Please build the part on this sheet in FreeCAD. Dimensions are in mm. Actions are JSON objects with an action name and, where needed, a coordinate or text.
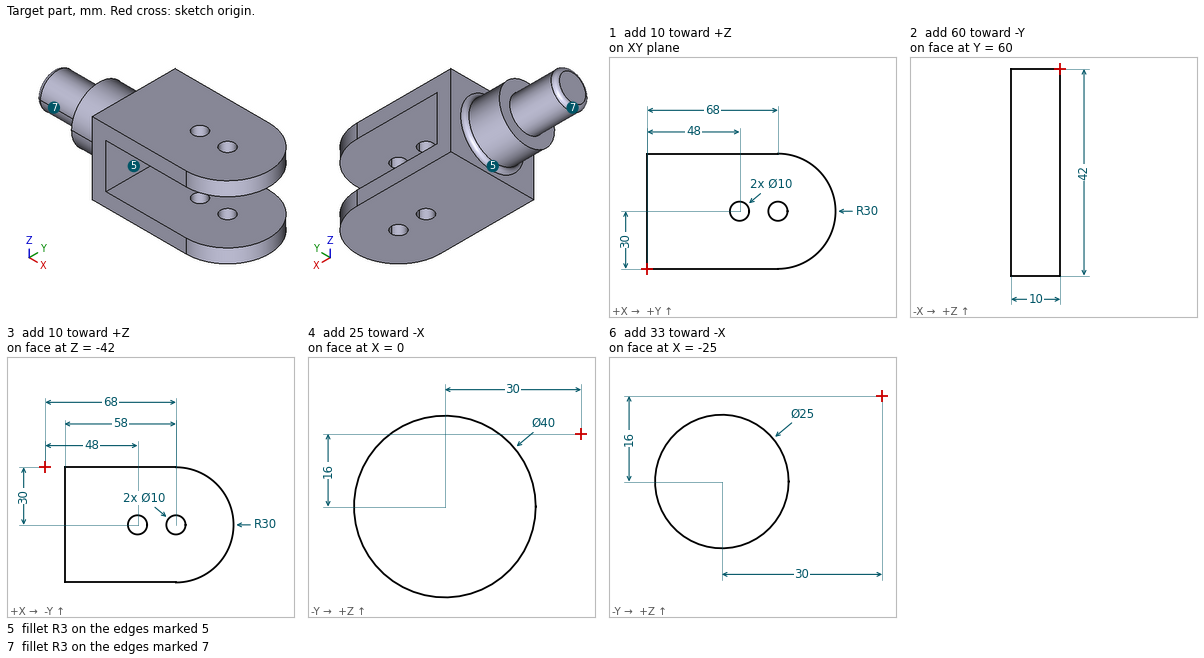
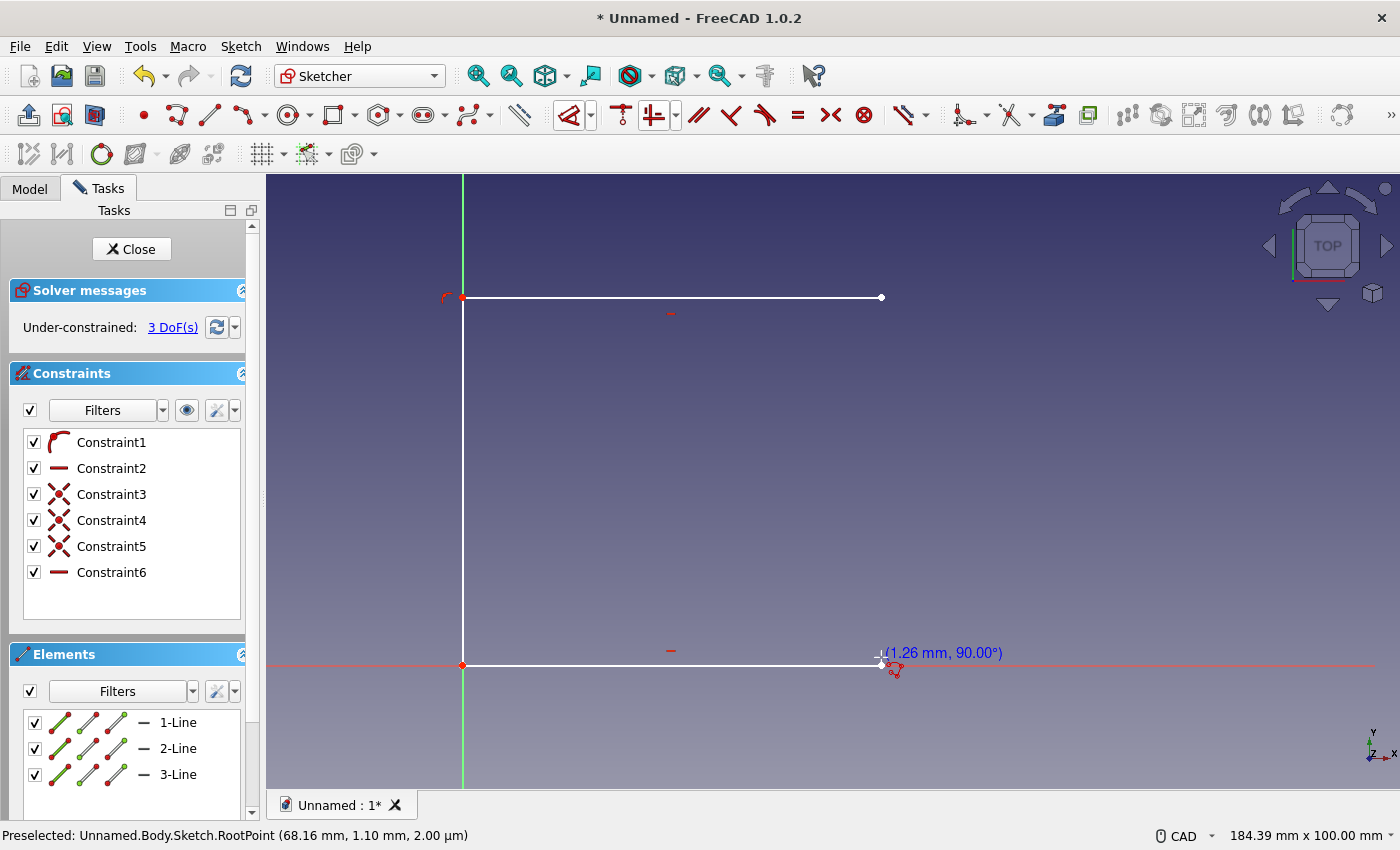
{"action": "key", "text": "g 3 a"}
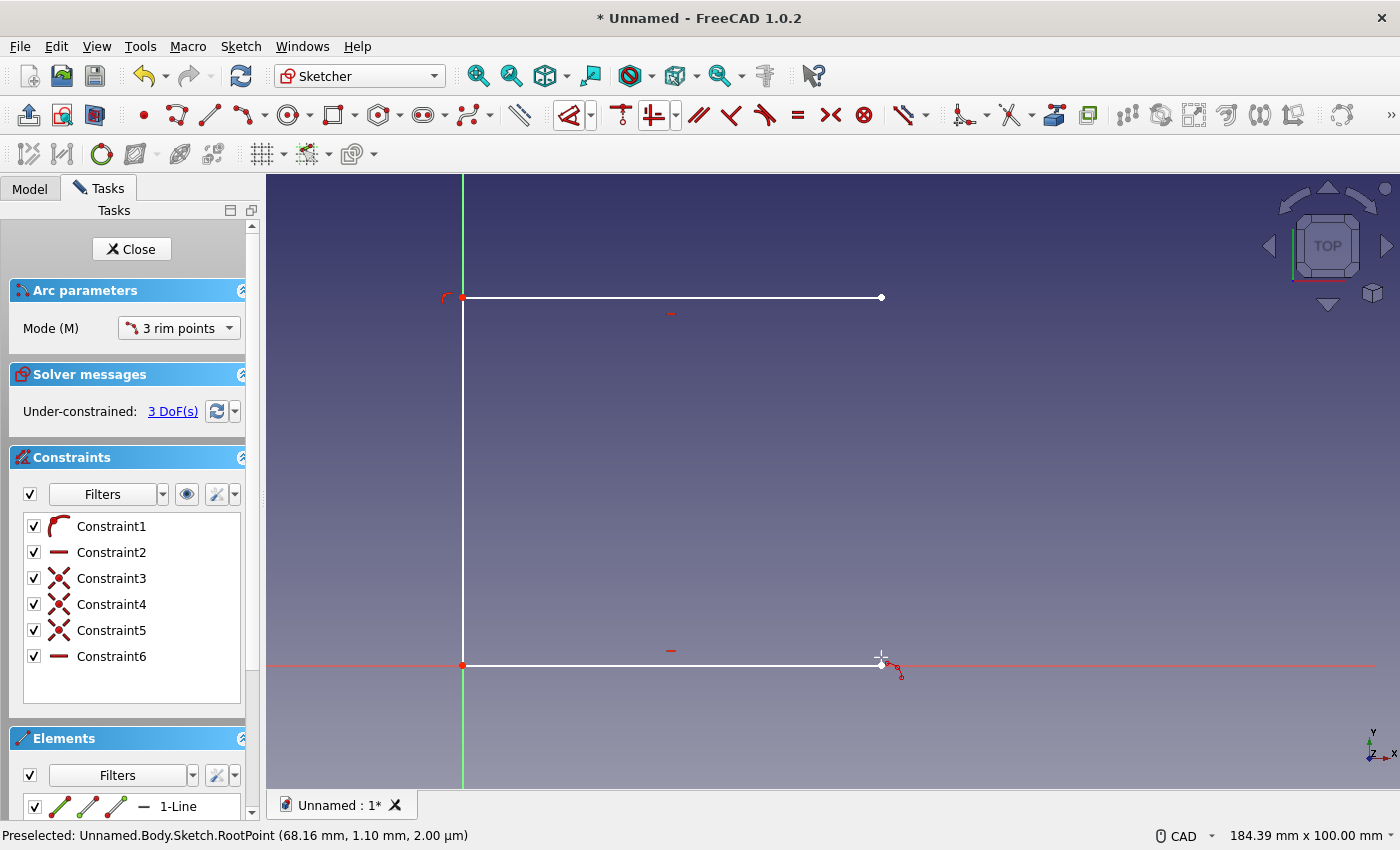
{"action": "left_click", "coordinate": [881, 666]}
{"action": "left_click", "coordinate": [881, 298]}
{"action": "left_click", "coordinate": [1066, 481]}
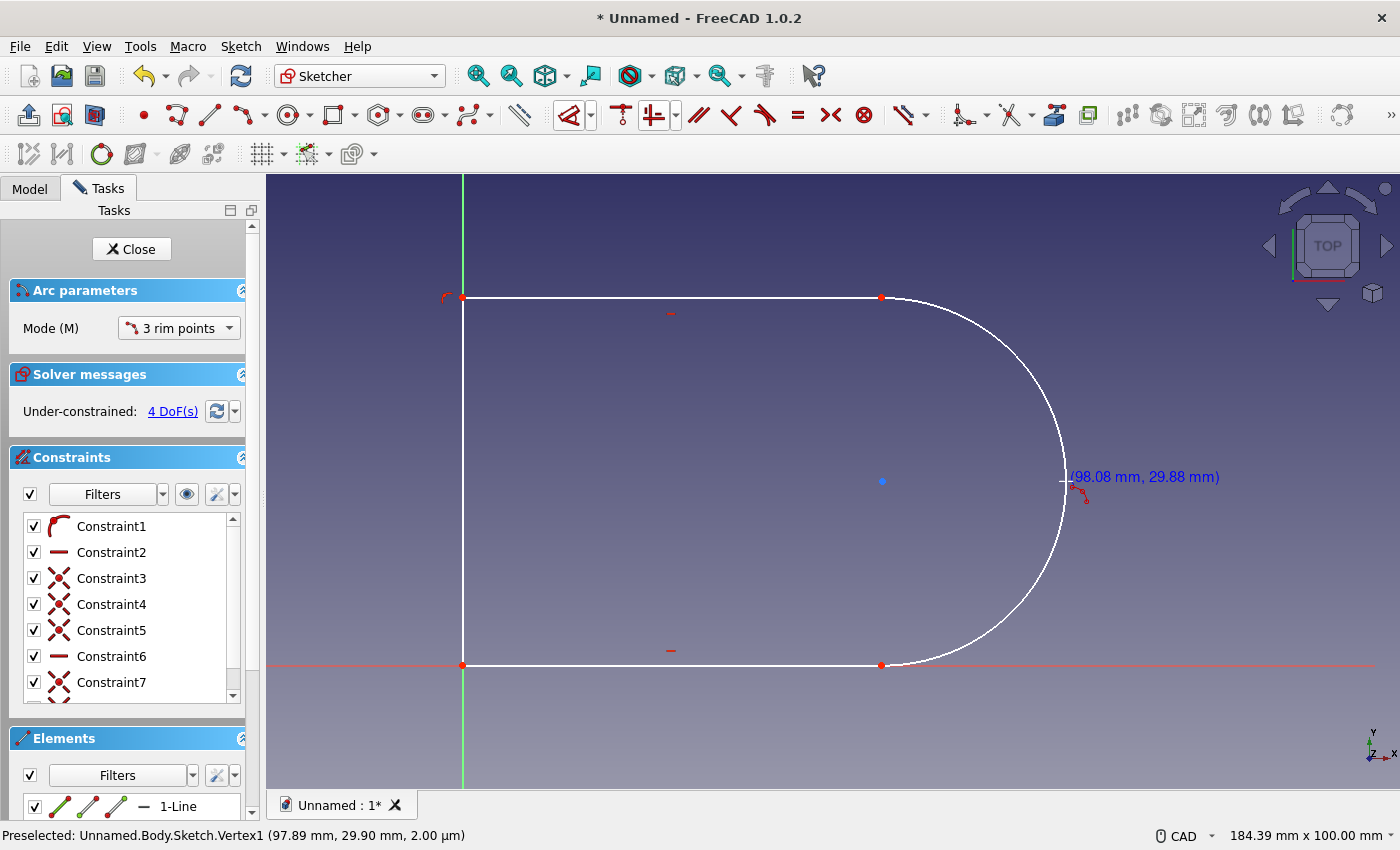
{"action": "key", "text": "g c"}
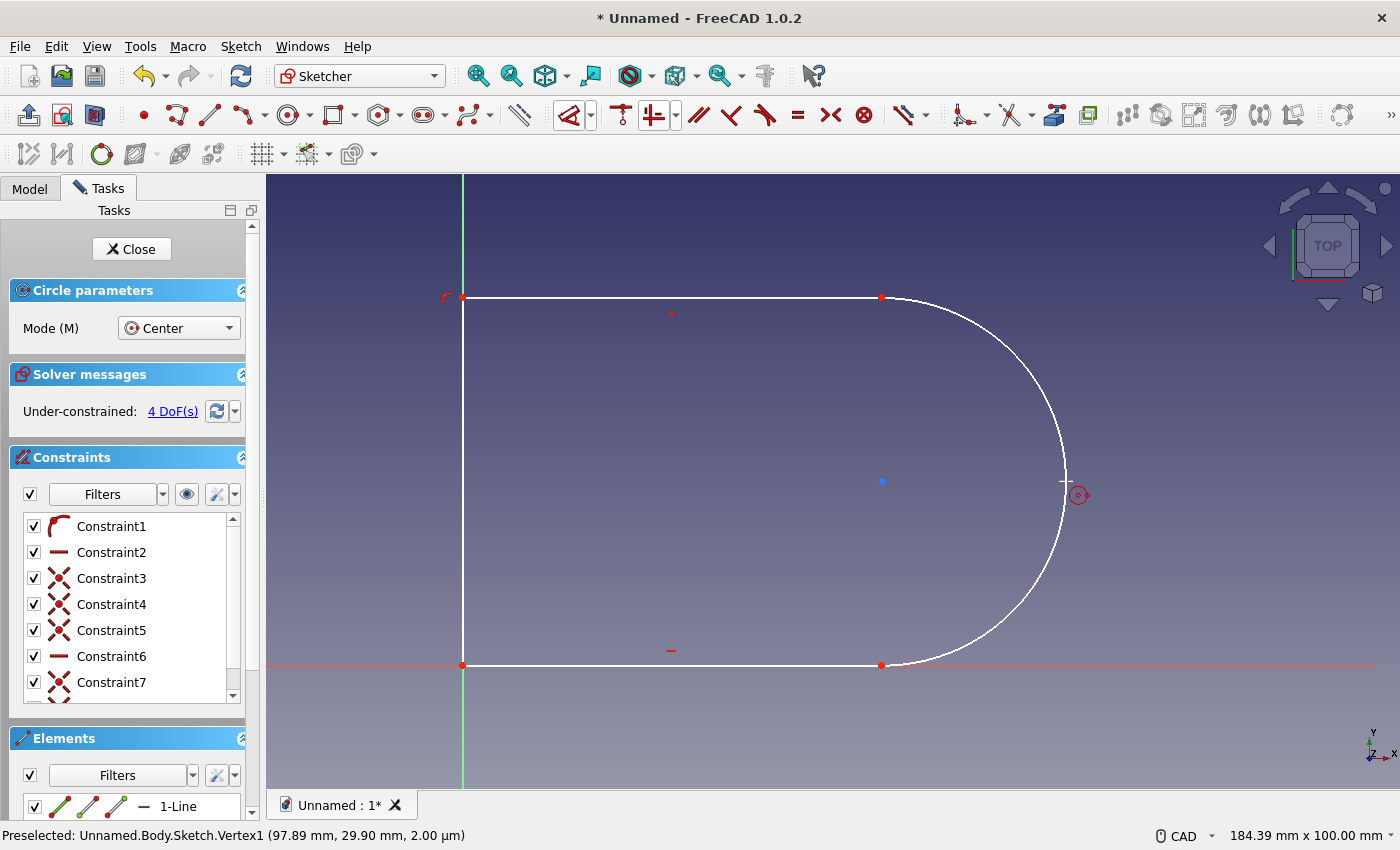
{"action": "left_click", "coordinate": [758, 481]}
{"action": "mouse_move", "coordinate": [780, 459]}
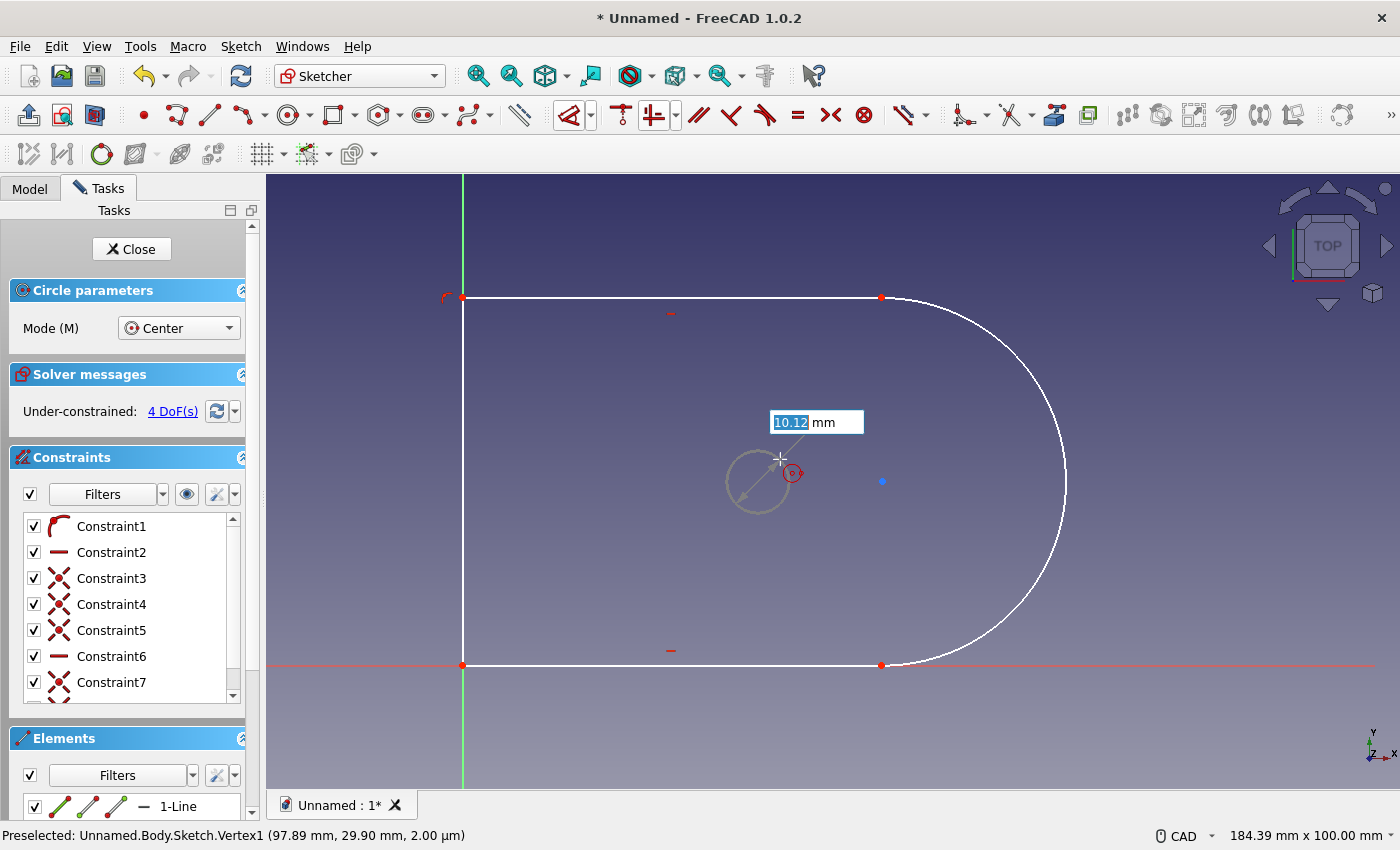
{"action": "type", "text": "10"}
{"action": "key", "text": "Return"}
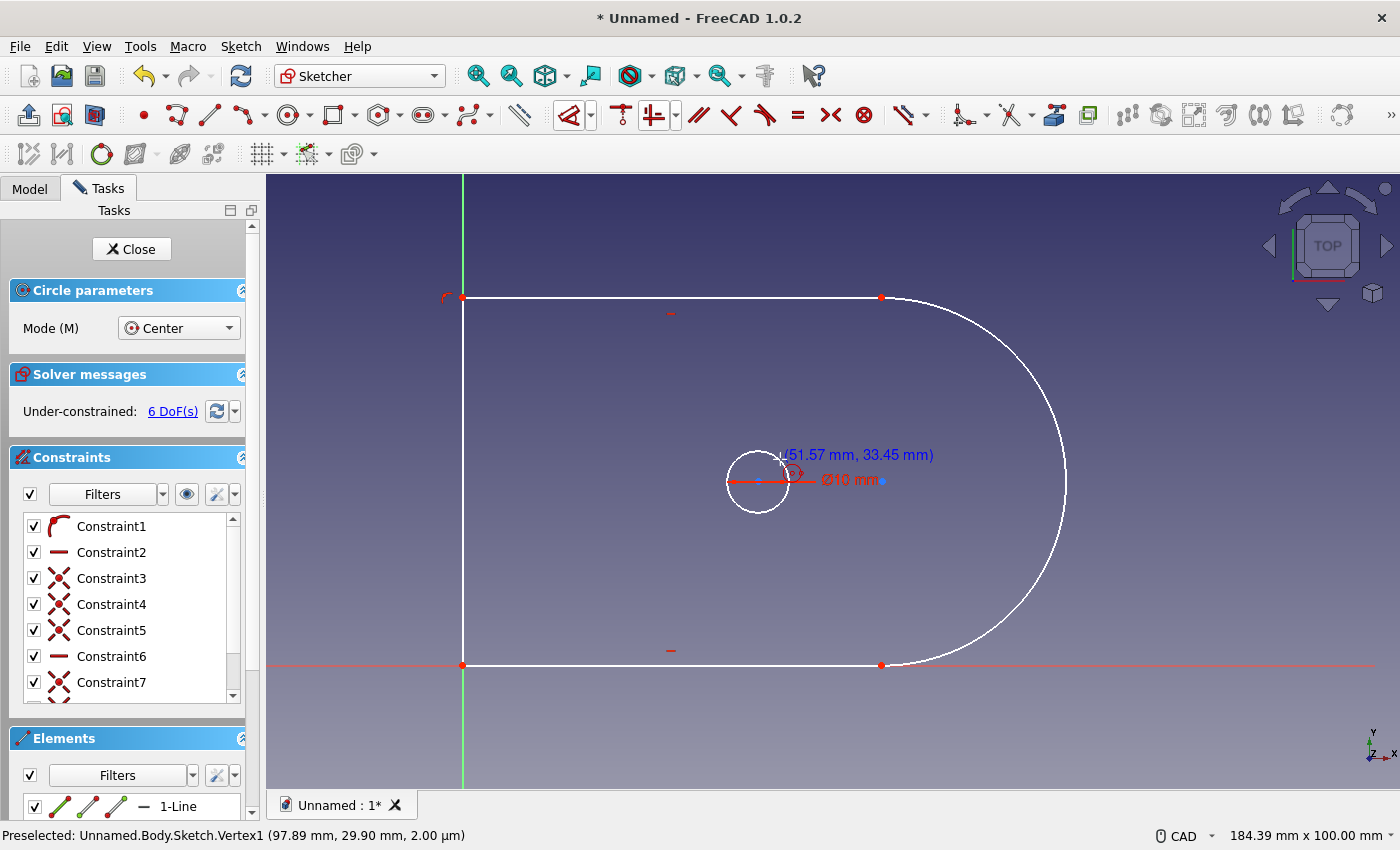
{"action": "left_click", "coordinate": [881, 481]}
{"action": "mouse_move", "coordinate": [903, 459]}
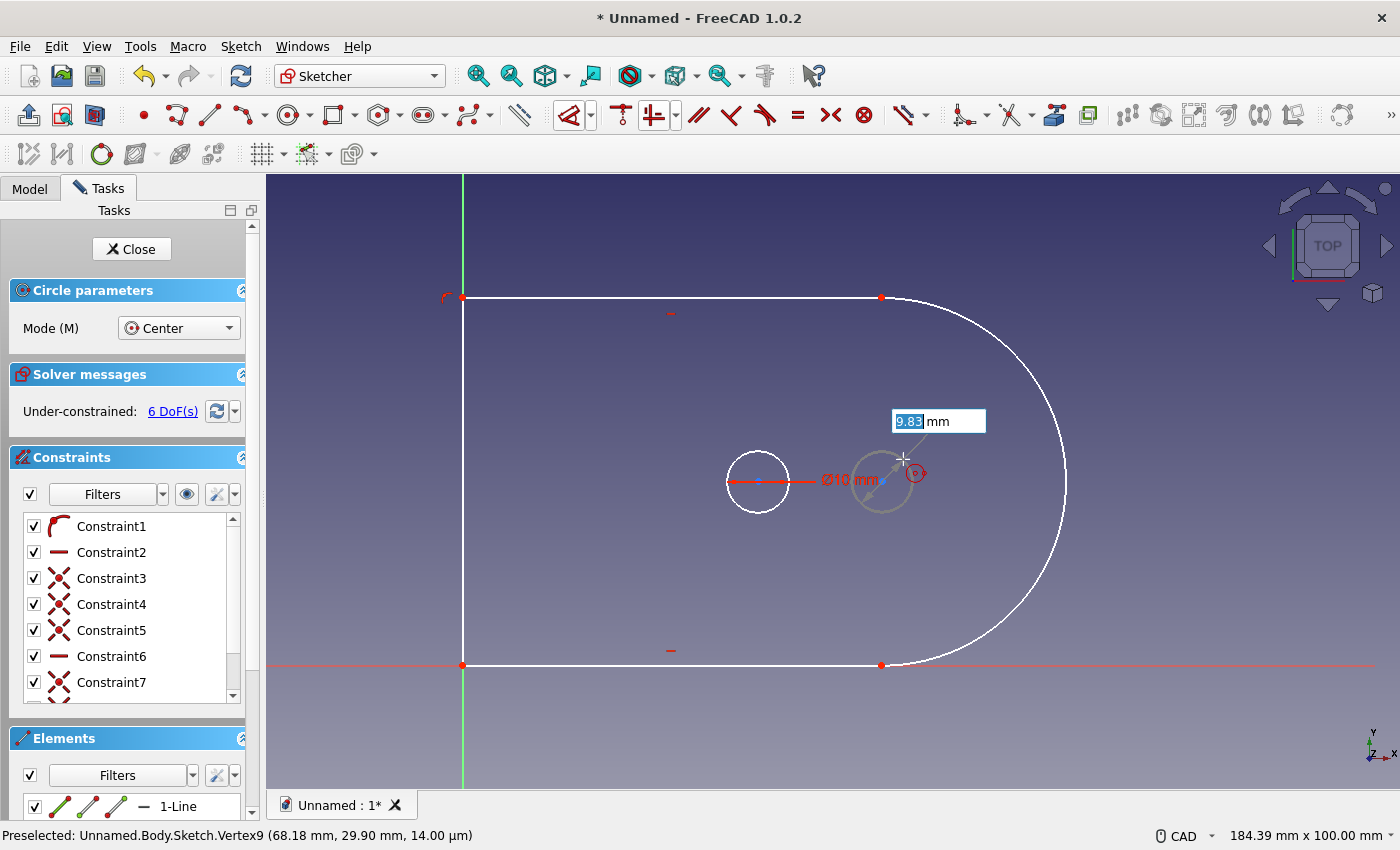
{"action": "type", "text": "10"}
{"action": "key", "text": "Return"}
{"action": "key", "text": "Escape"}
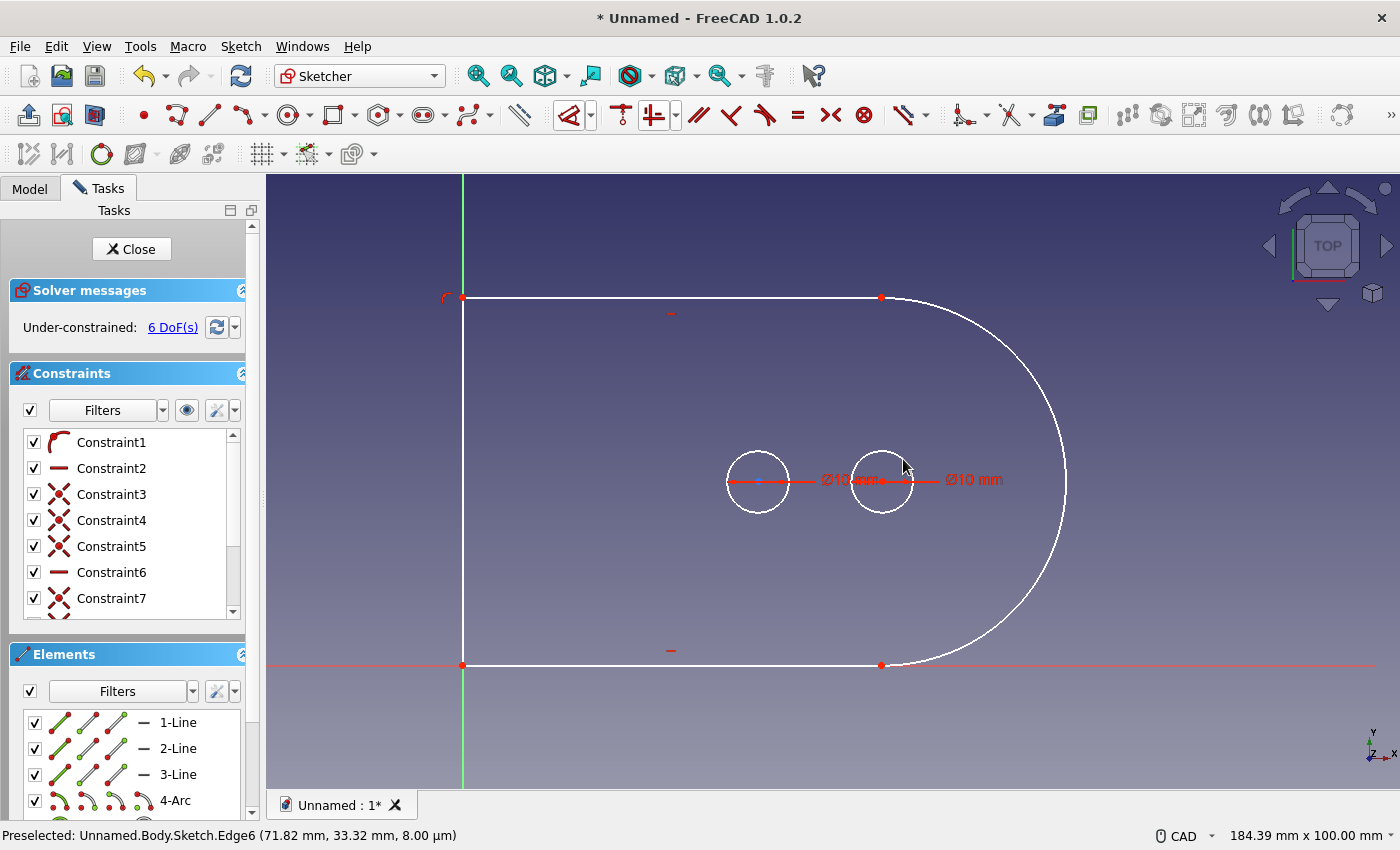
{"action": "left_click", "coordinate": [756, 298]}